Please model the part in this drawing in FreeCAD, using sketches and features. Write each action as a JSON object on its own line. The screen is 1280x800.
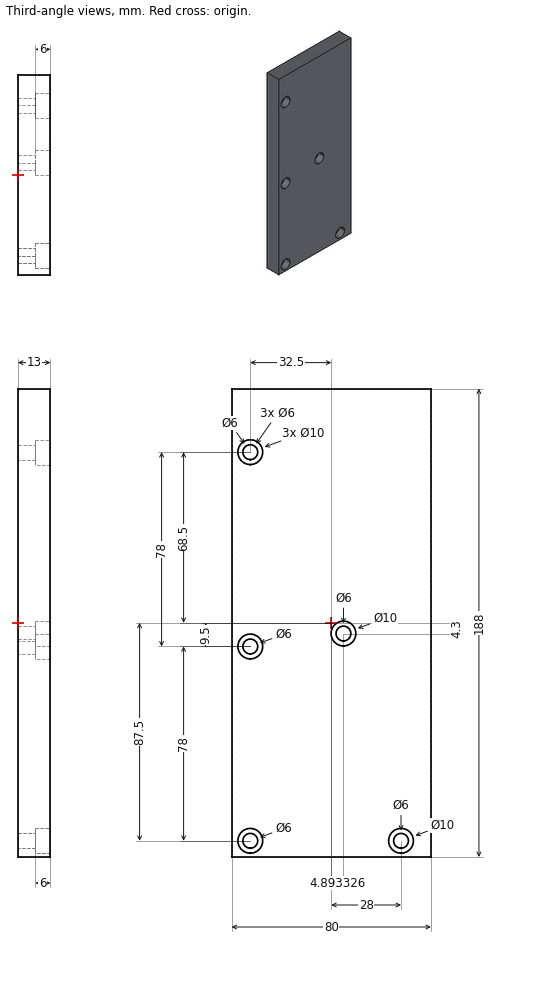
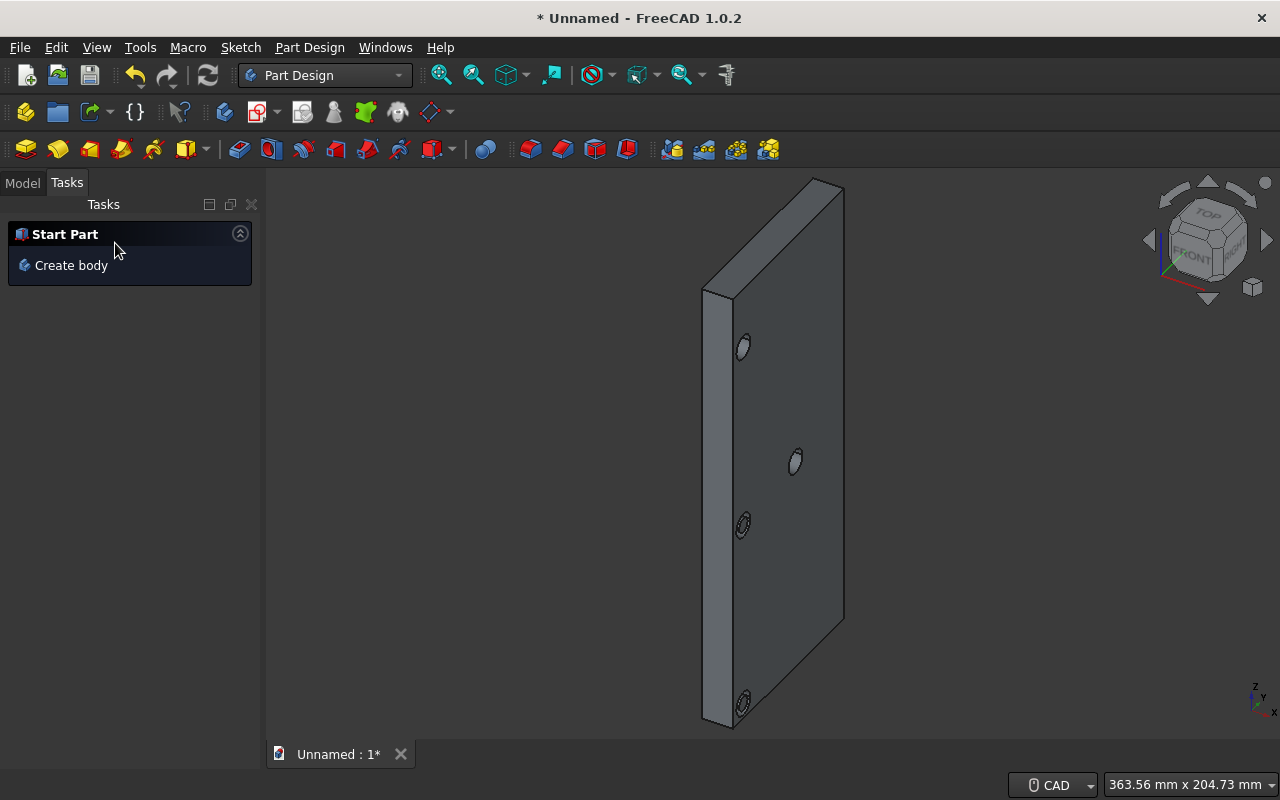
{"action": "left_click", "coordinate": [789, 580]}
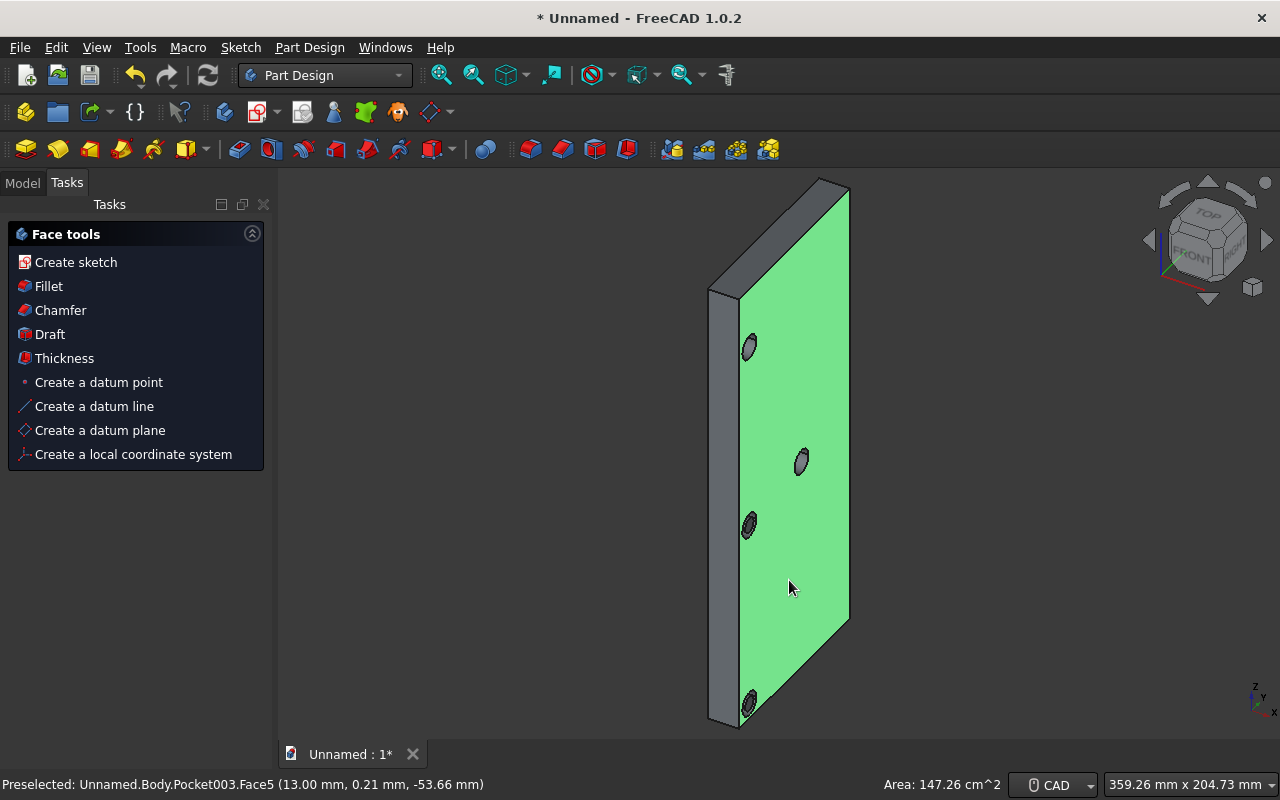
{"action": "left_click", "coordinate": [258, 112]}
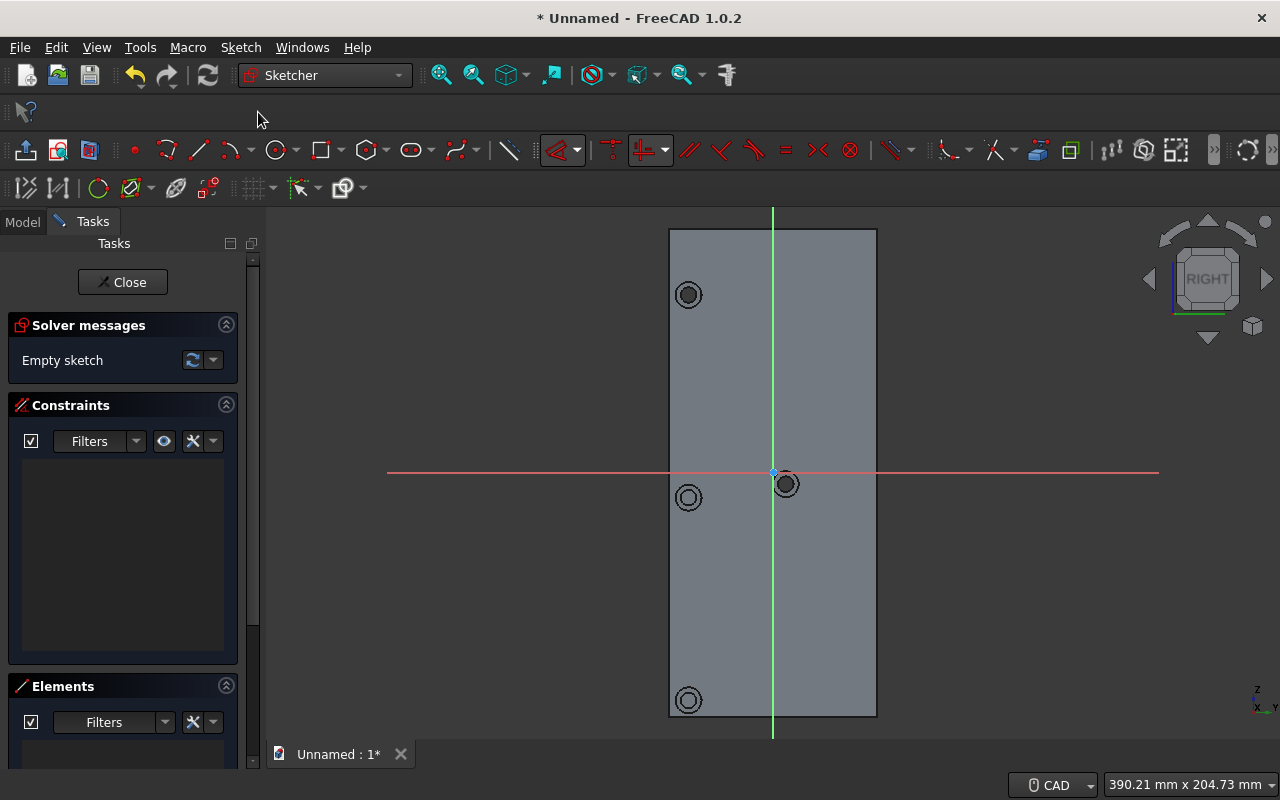
{"action": "scroll", "coordinate": [688, 499], "scroll_direction": "up", "scroll_amount": 15}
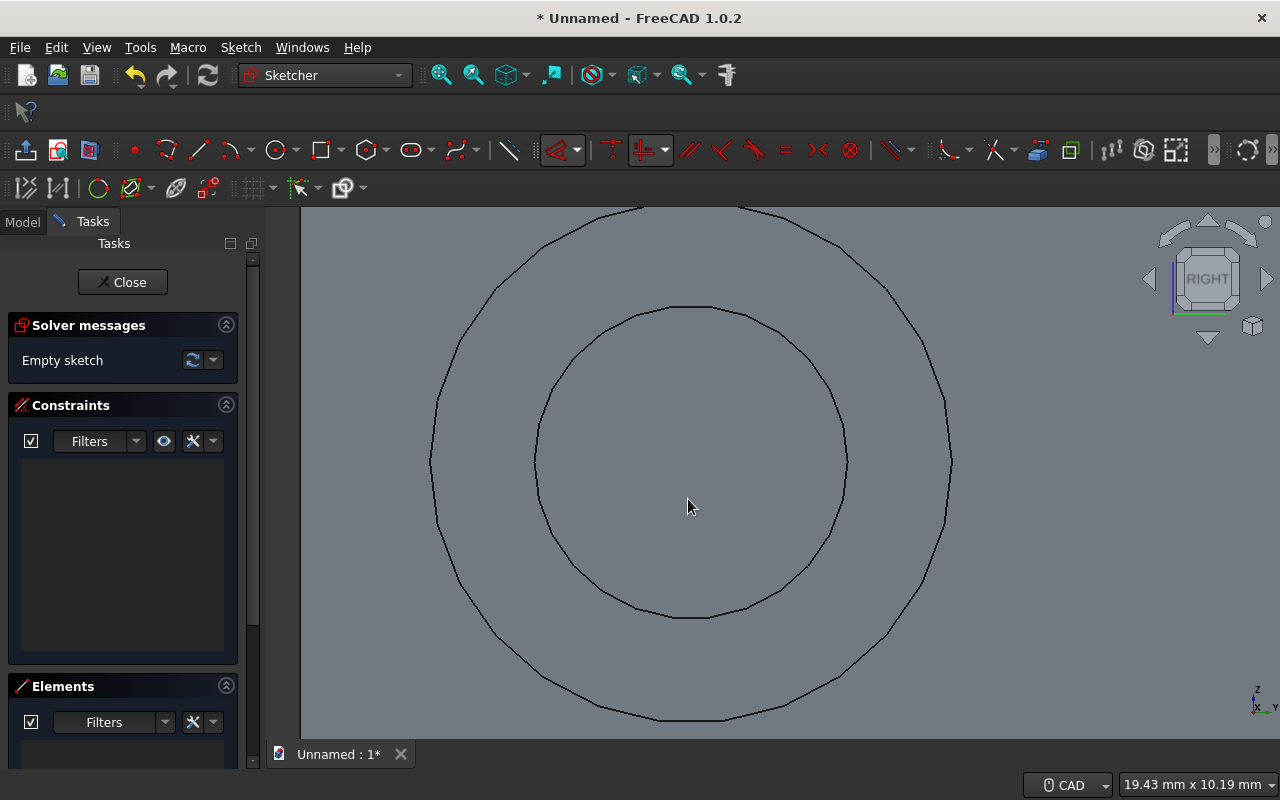
{"action": "left_click", "coordinate": [276, 150]}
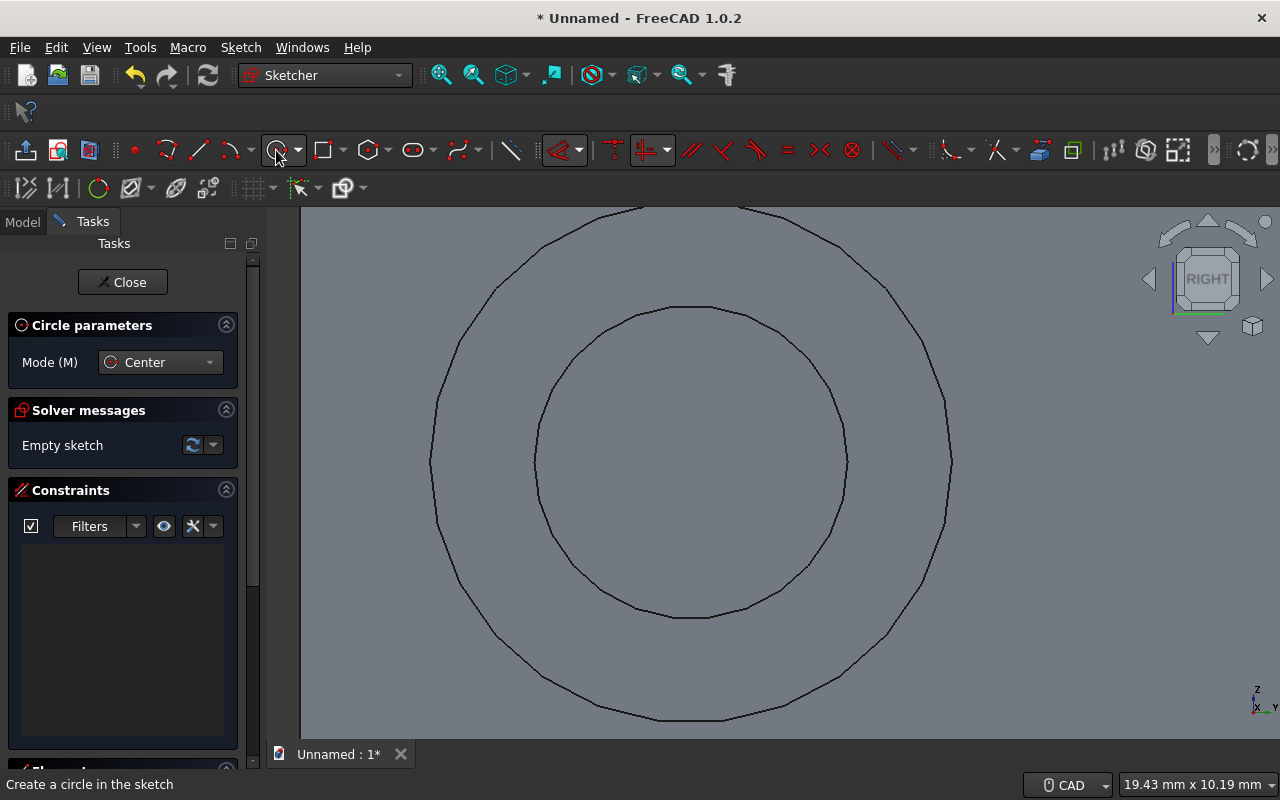
{"action": "left_click", "coordinate": [691, 462]}
{"action": "left_click", "coordinate": [802, 351]}
{"action": "key", "text": "Escape"}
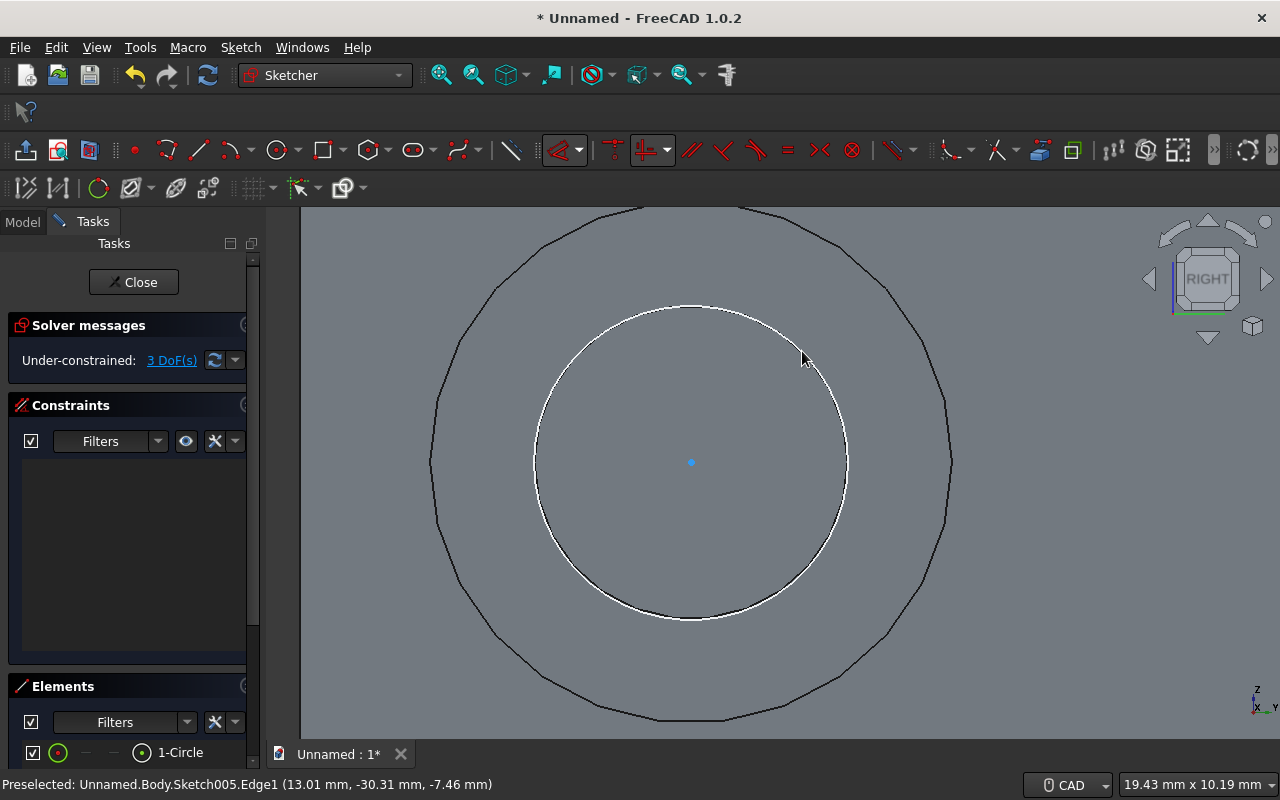
{"action": "left_click", "coordinate": [802, 352]}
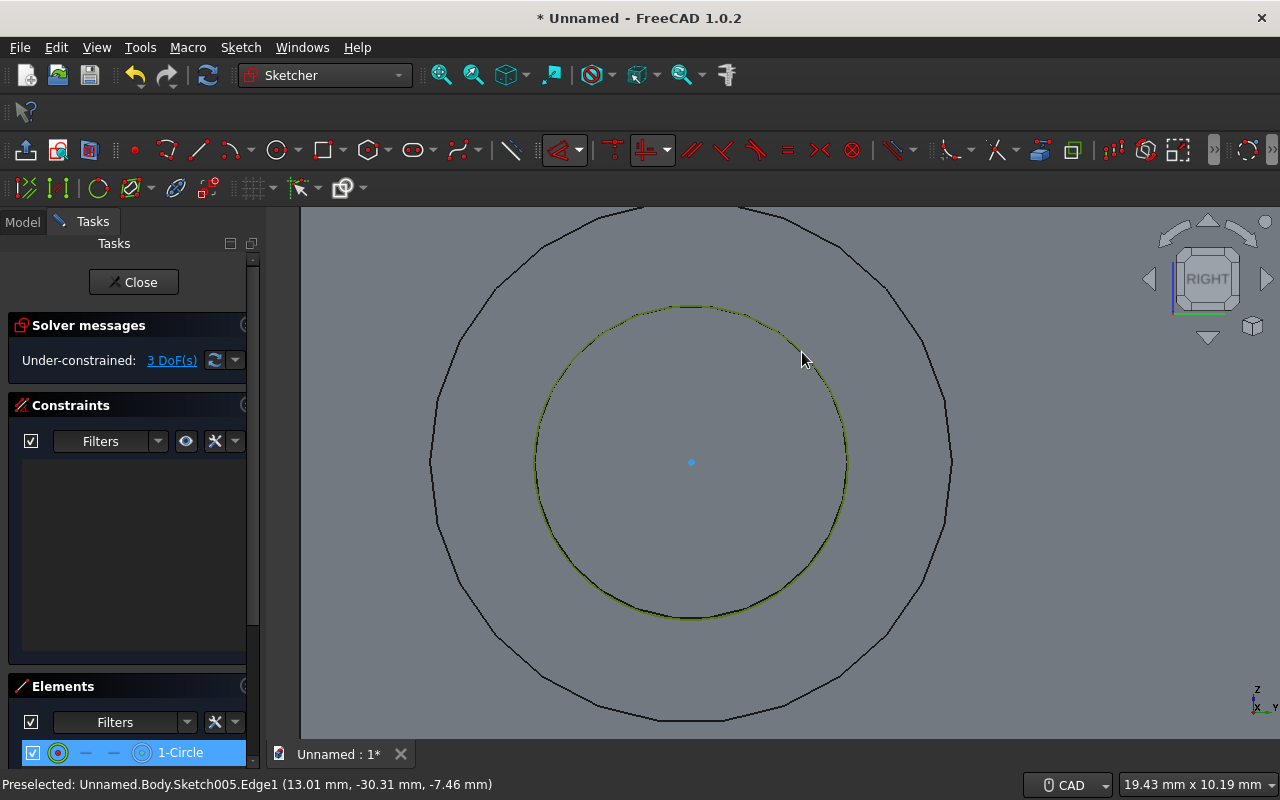
{"action": "key", "text": "k o"}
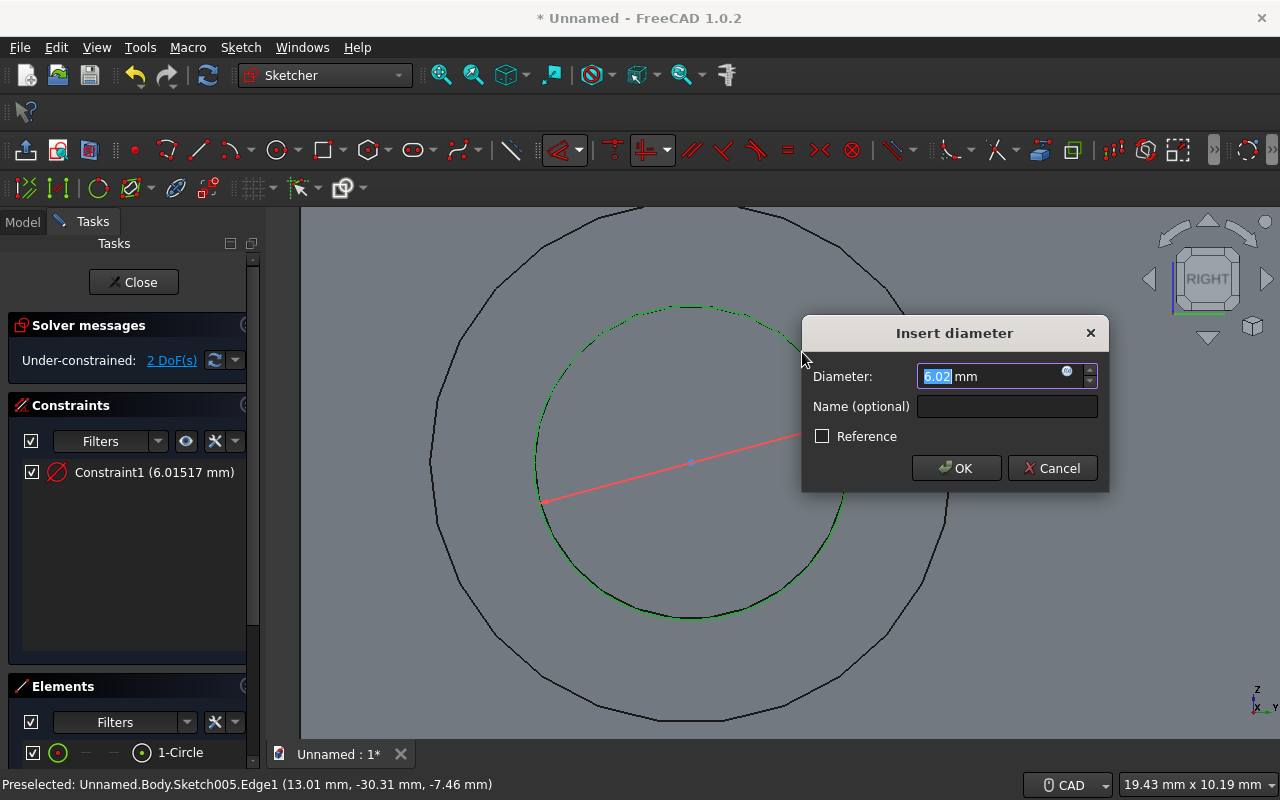
{"action": "type", "text": "6"}
{"action": "key", "text": "Return"}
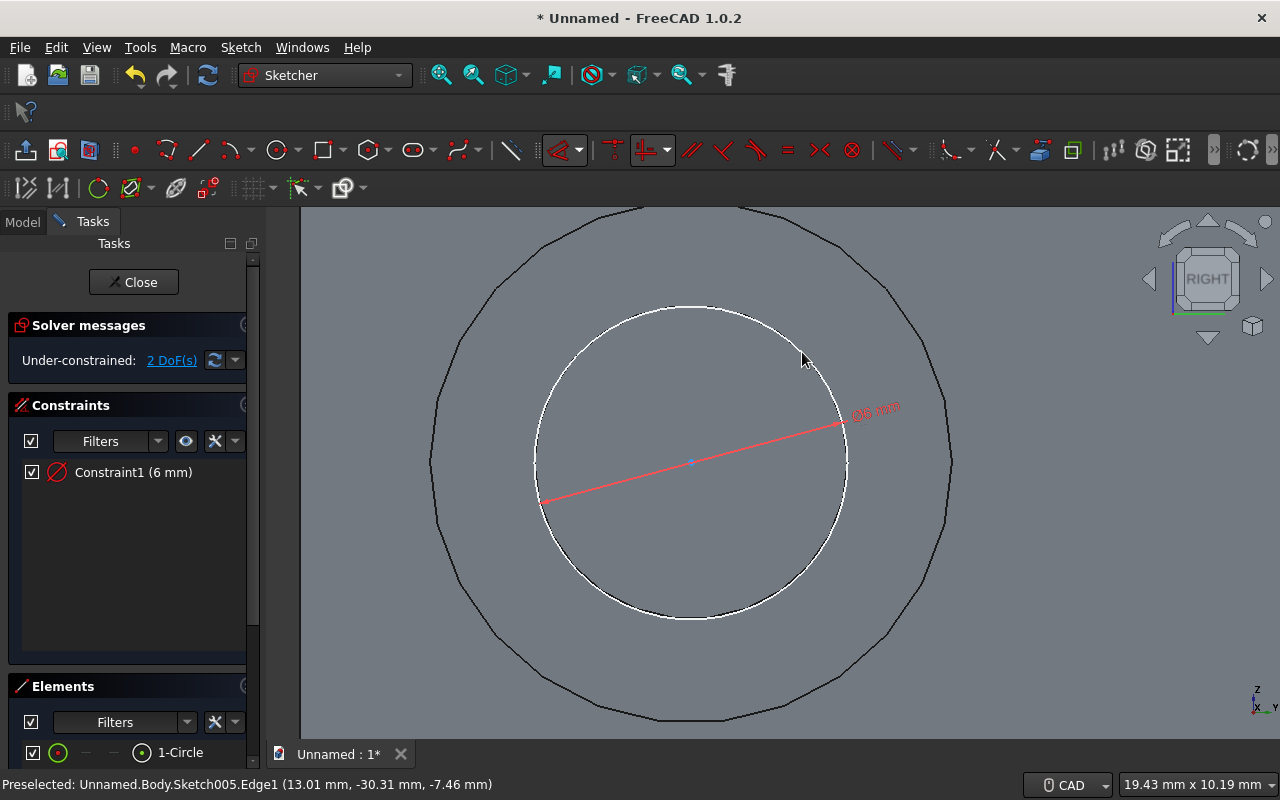
{"action": "left_click", "coordinate": [691, 463]}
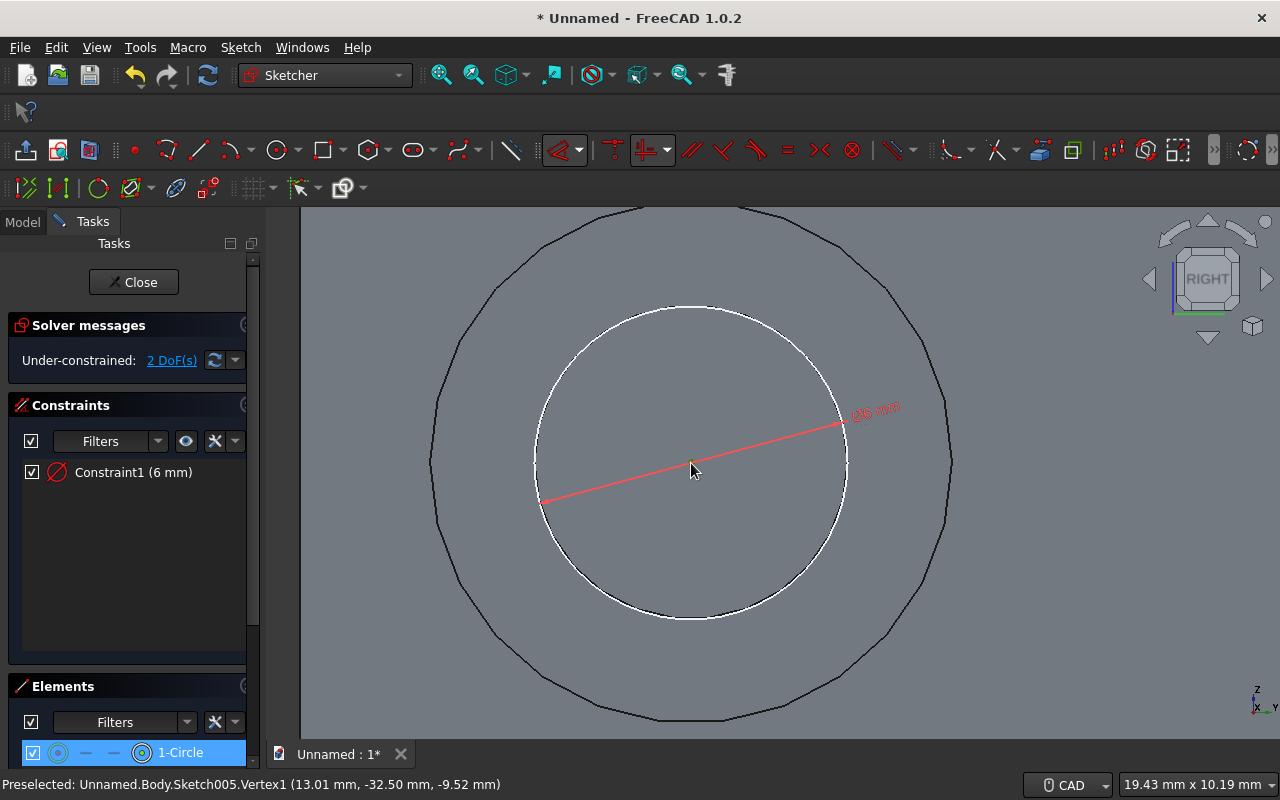
{"action": "left_click", "coordinate": [582, 150]}